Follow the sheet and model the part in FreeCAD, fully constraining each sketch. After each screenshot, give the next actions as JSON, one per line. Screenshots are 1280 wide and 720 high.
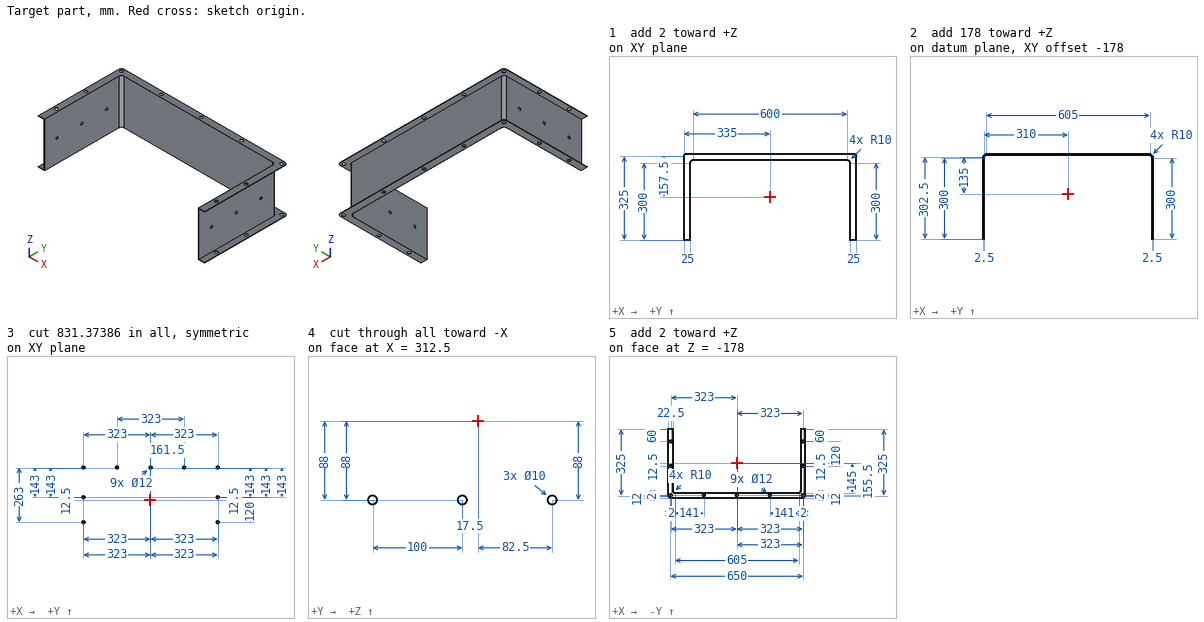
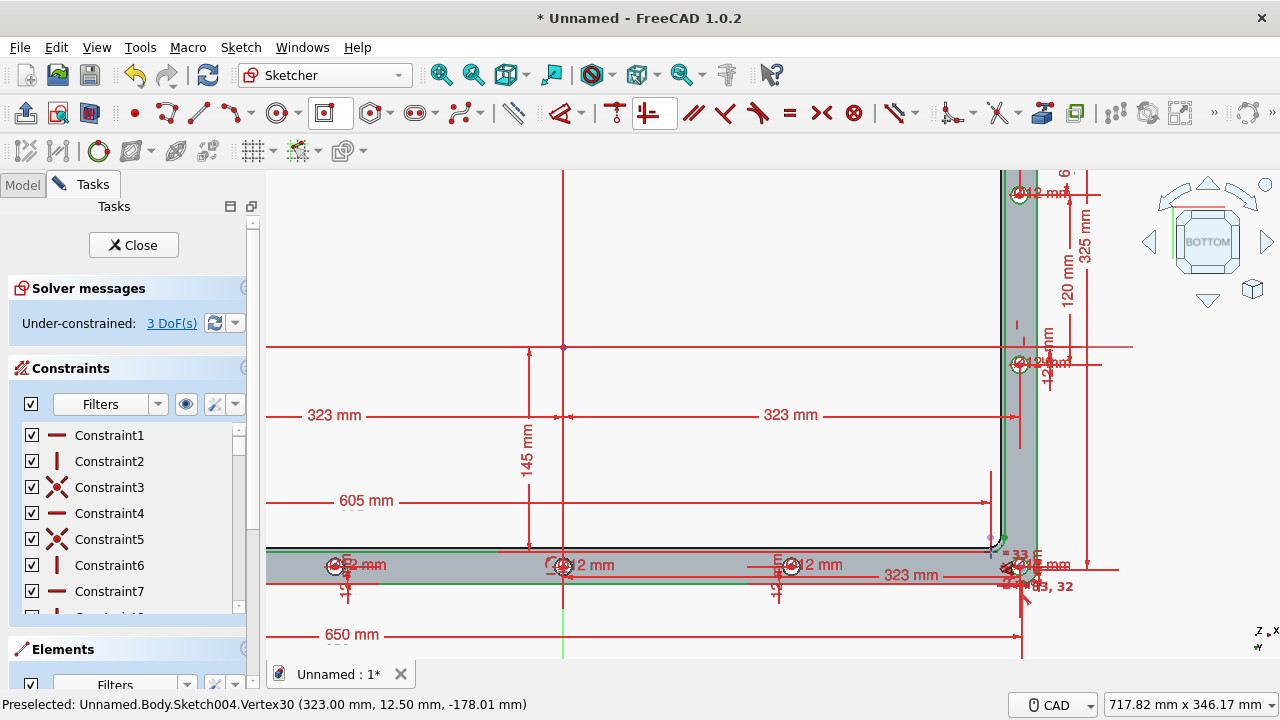
{"action": "left_click", "coordinate": [991, 552]}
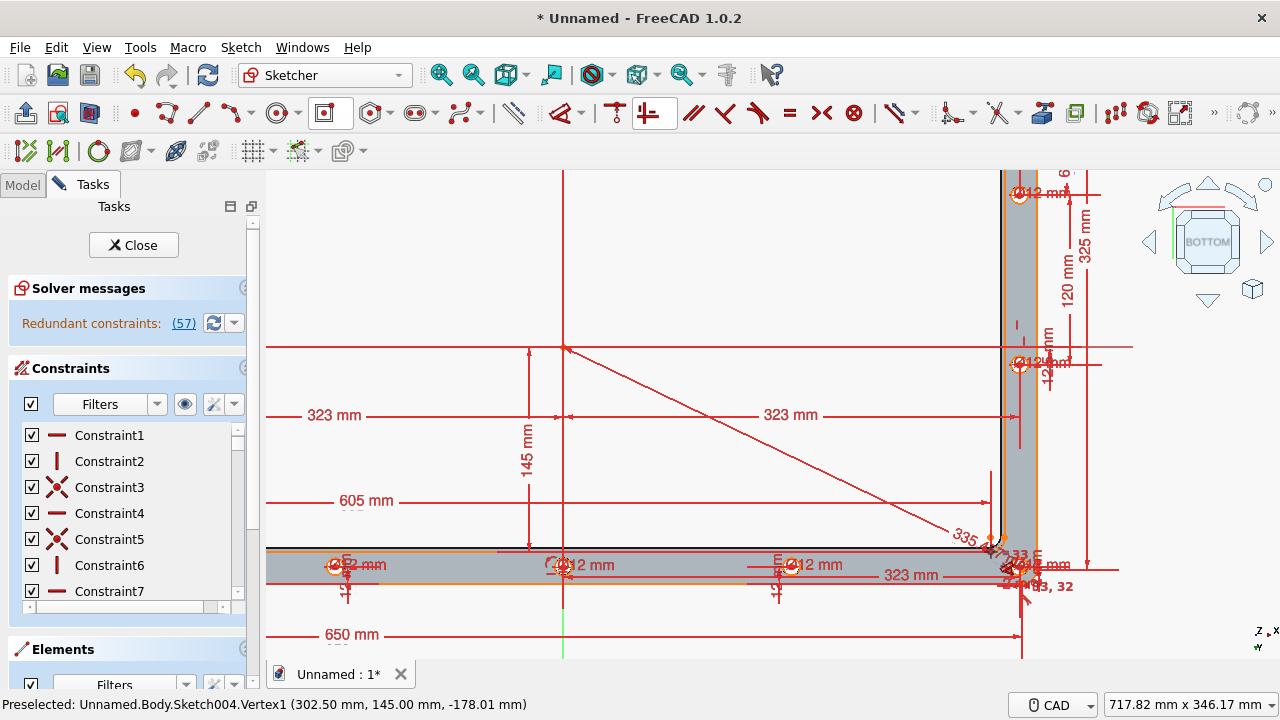
{"action": "left_click", "coordinate": [792, 567]}
{"action": "left_click", "coordinate": [891, 601]}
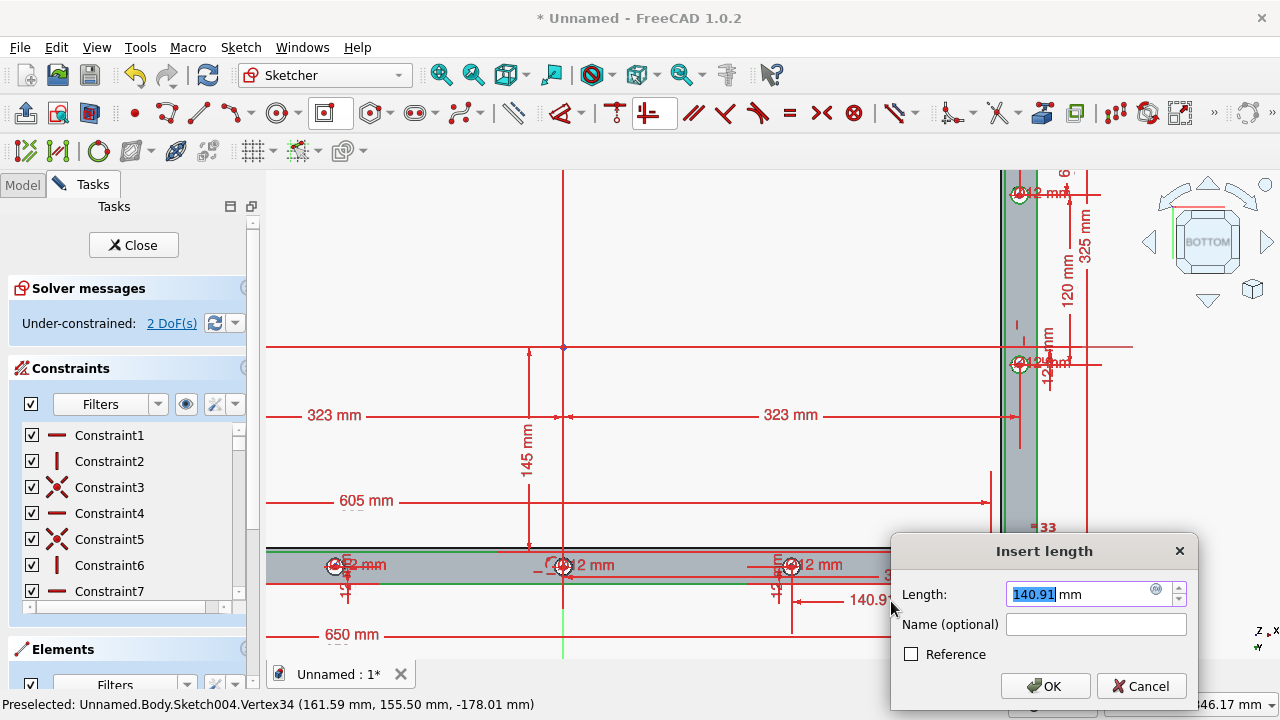
{"action": "type", "text": "141"}
{"action": "key", "text": "Return"}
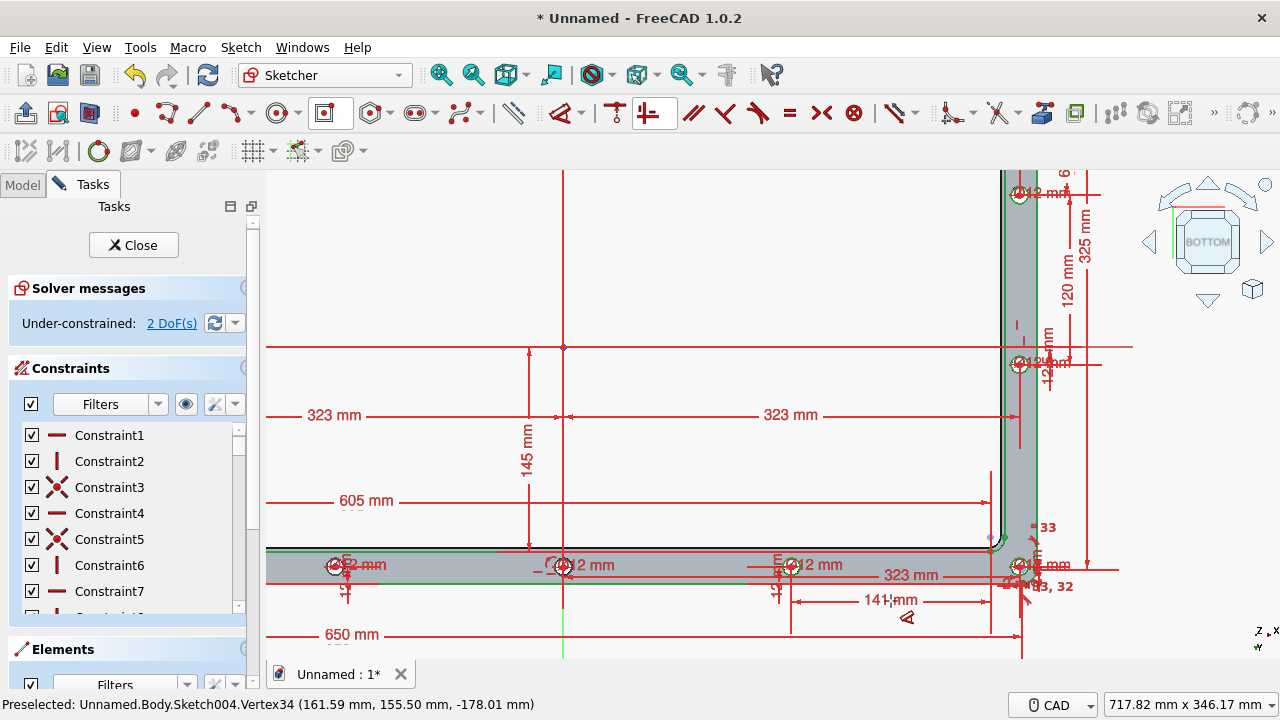
{"action": "scroll", "coordinate": [991, 551], "scroll_direction": "down", "scroll_amount": 2}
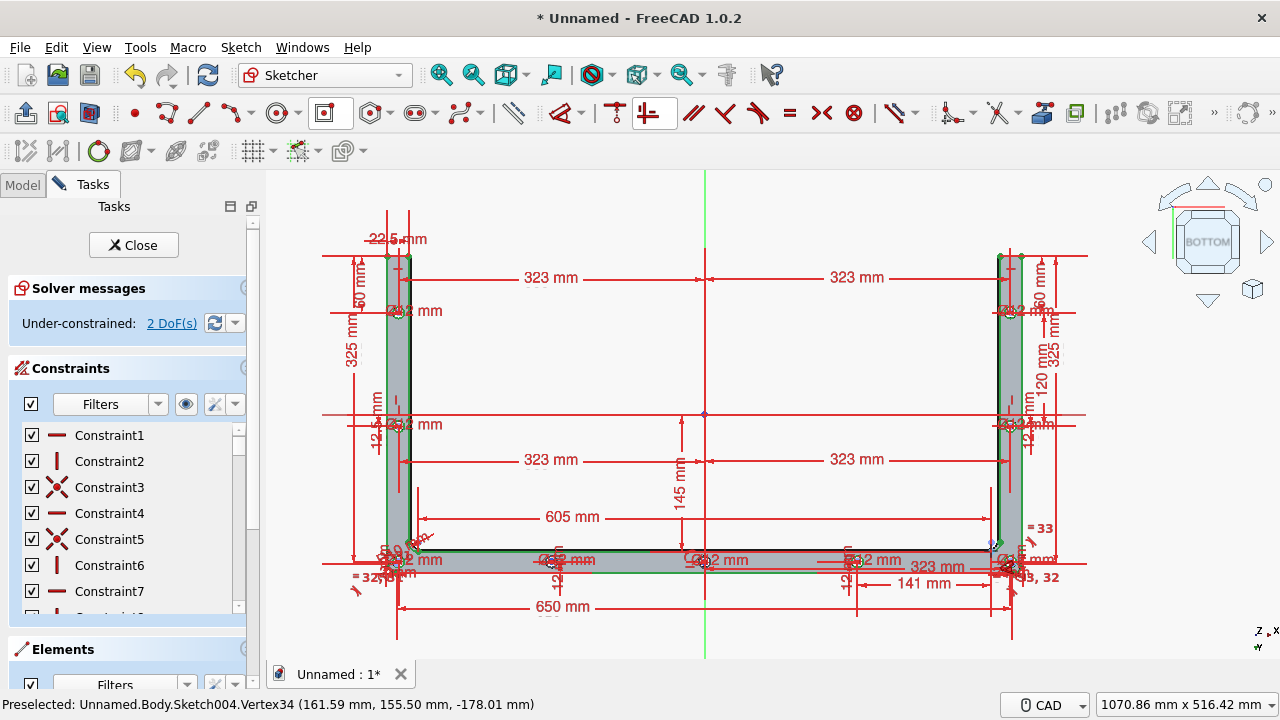
{"action": "scroll", "coordinate": [418, 552], "scroll_direction": "up", "scroll_amount": 2}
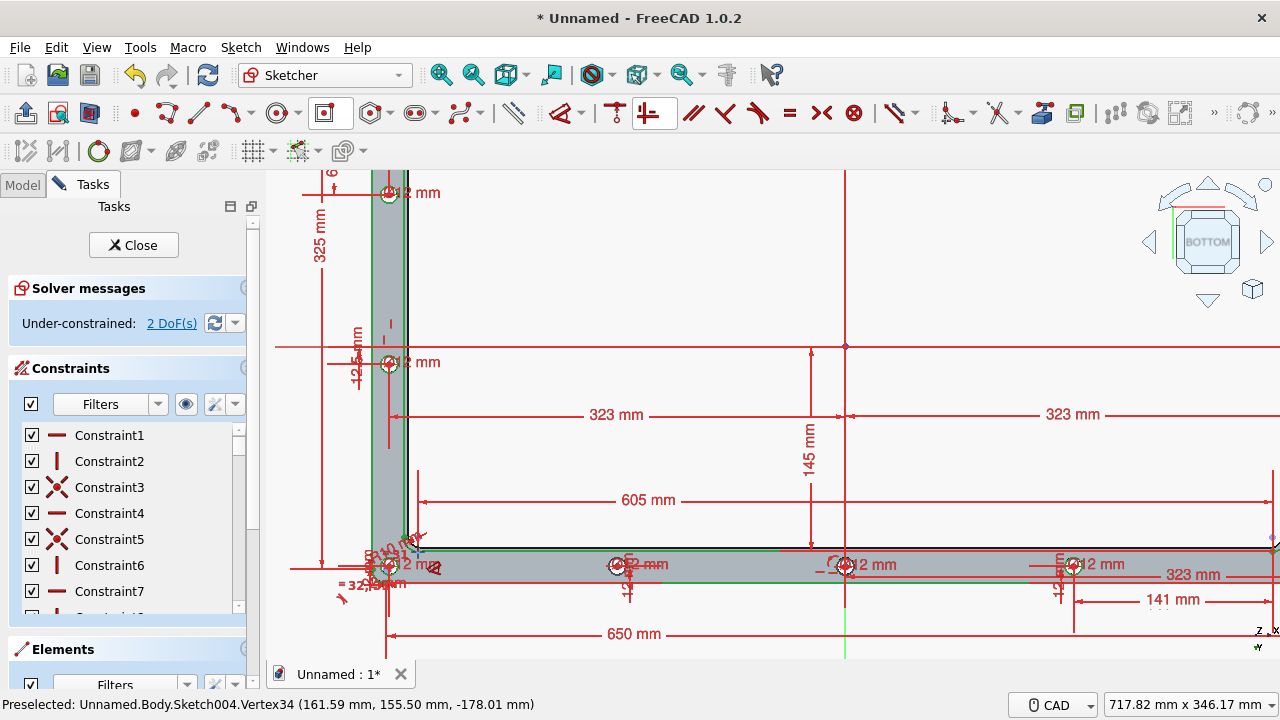
{"action": "left_click", "coordinate": [418, 551]}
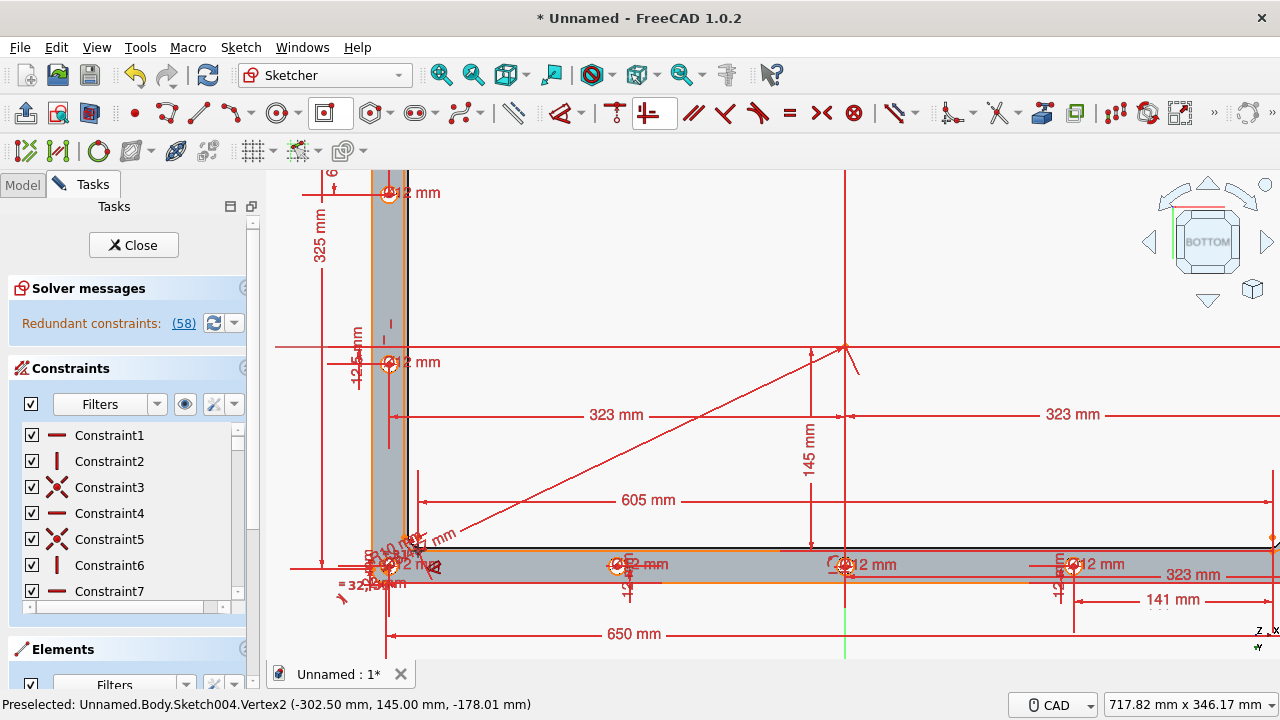
{"action": "left_click", "coordinate": [617, 566]}
{"action": "left_click", "coordinate": [518, 600]}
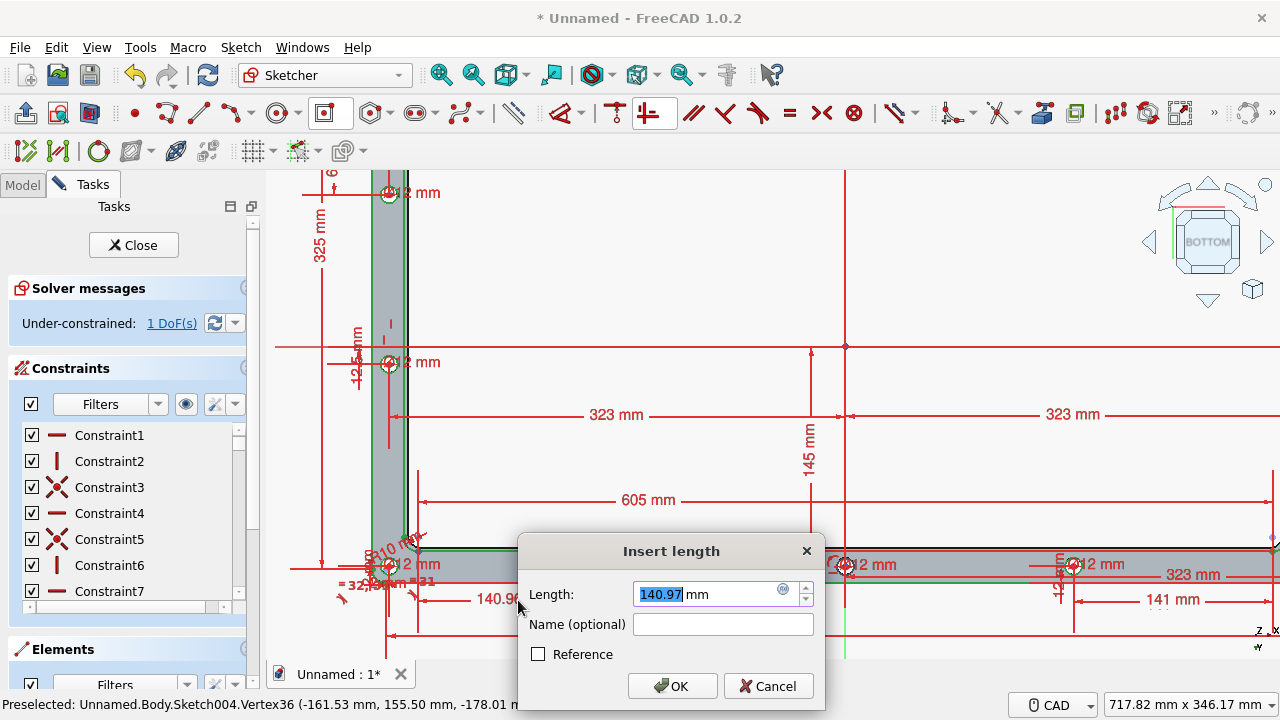
{"action": "type", "text": "141"}
{"action": "key", "text": "Return"}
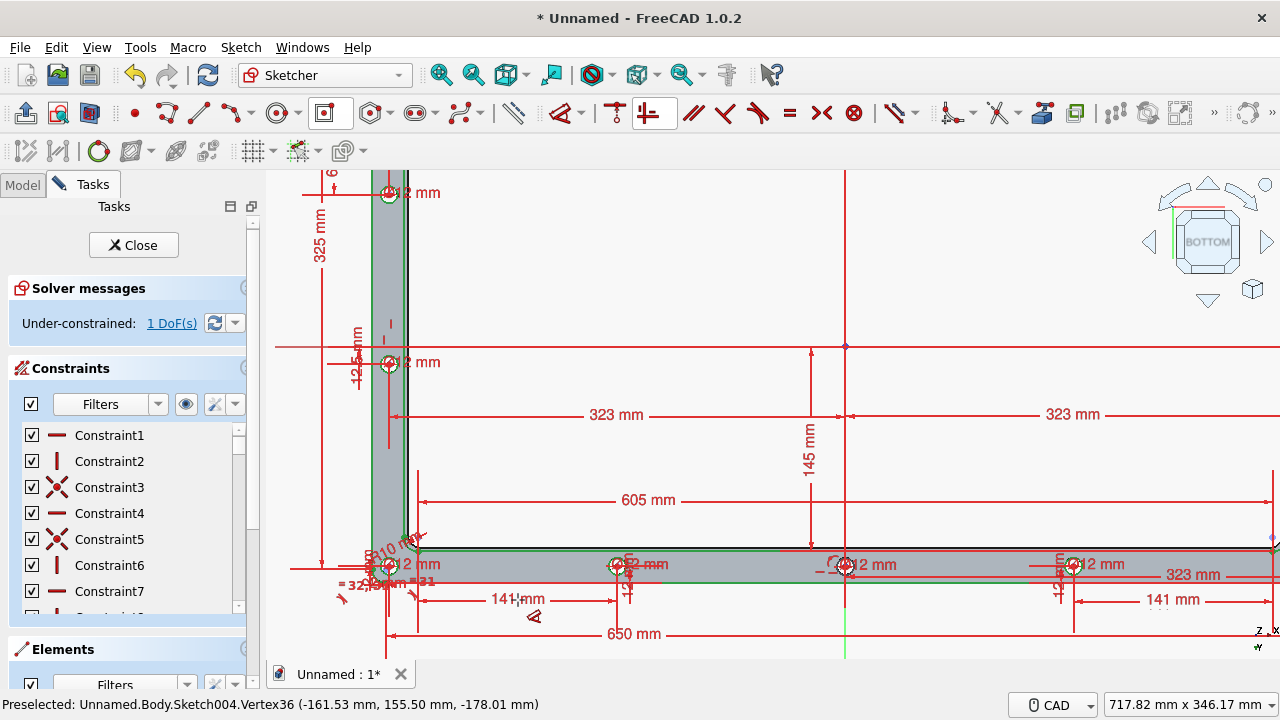
{"action": "left_click", "coordinate": [845, 567]}
{"action": "left_click", "coordinate": [879, 406]}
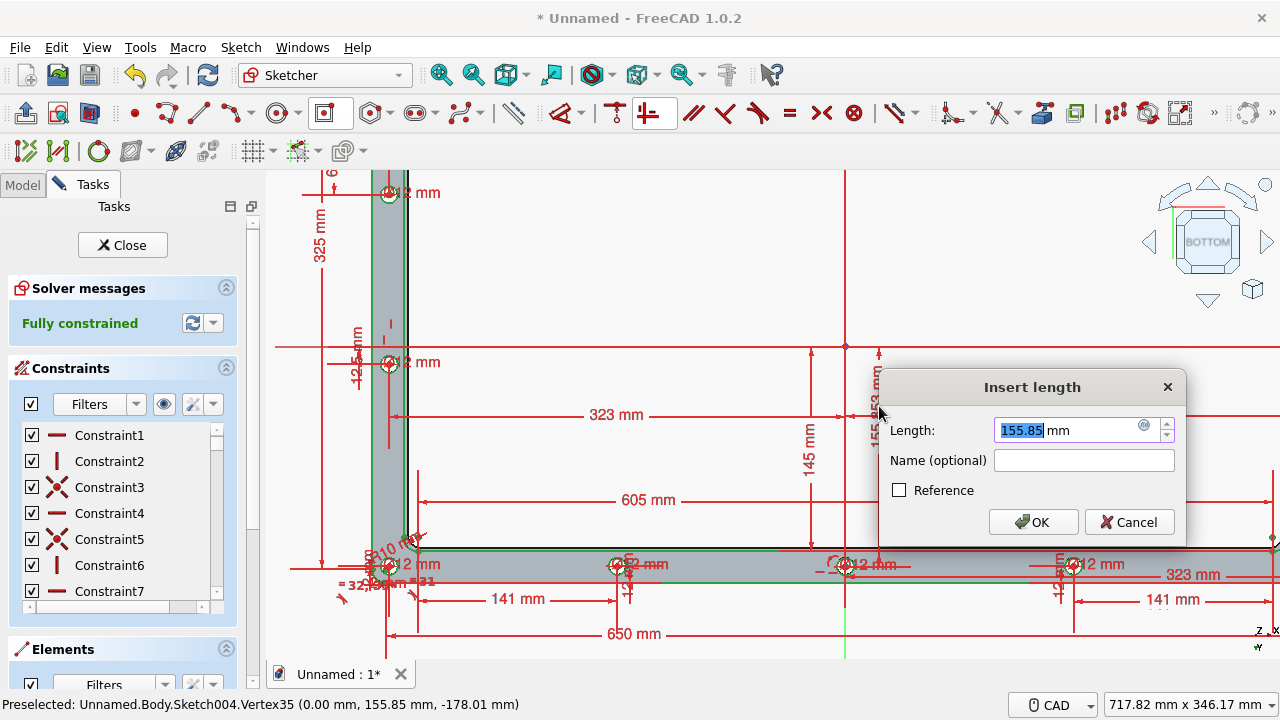
{"action": "type", "text": "155.5"}
{"action": "key", "text": "Return"}
{"action": "key", "text": "Escape"}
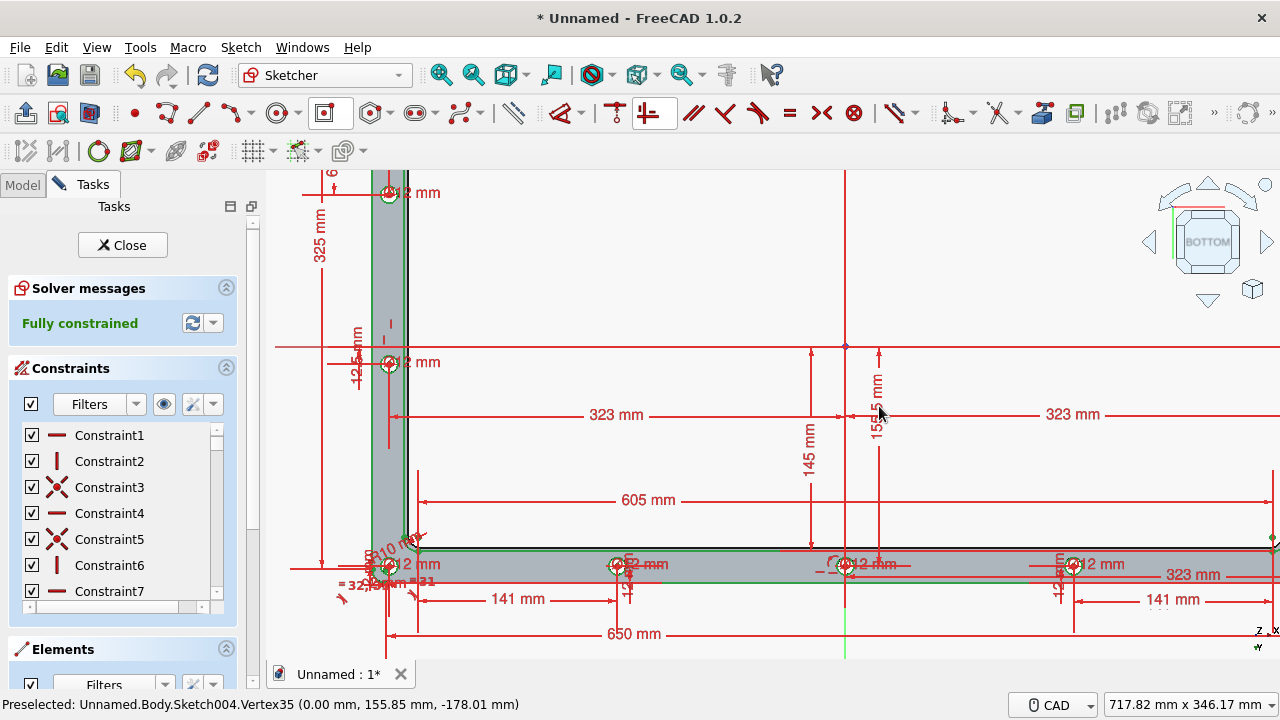
{"action": "left_click", "coordinate": [123, 245]}